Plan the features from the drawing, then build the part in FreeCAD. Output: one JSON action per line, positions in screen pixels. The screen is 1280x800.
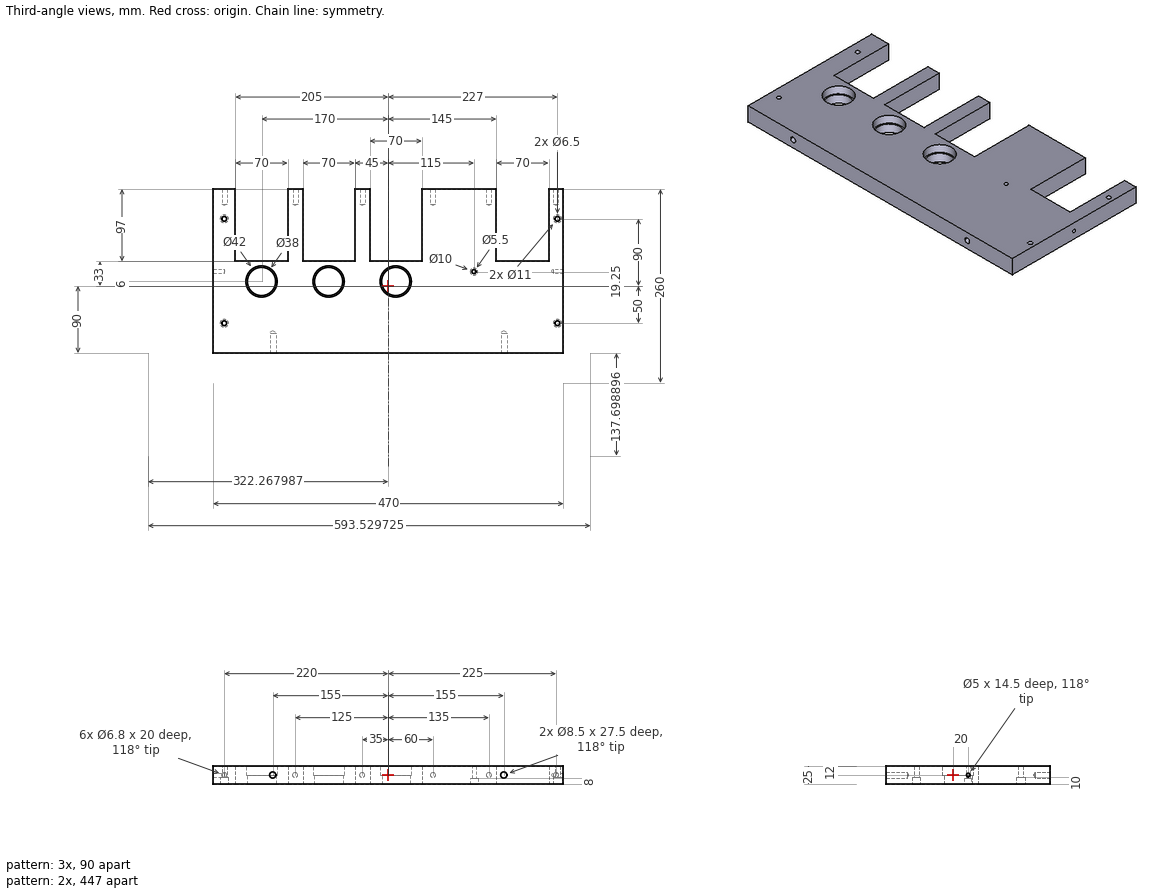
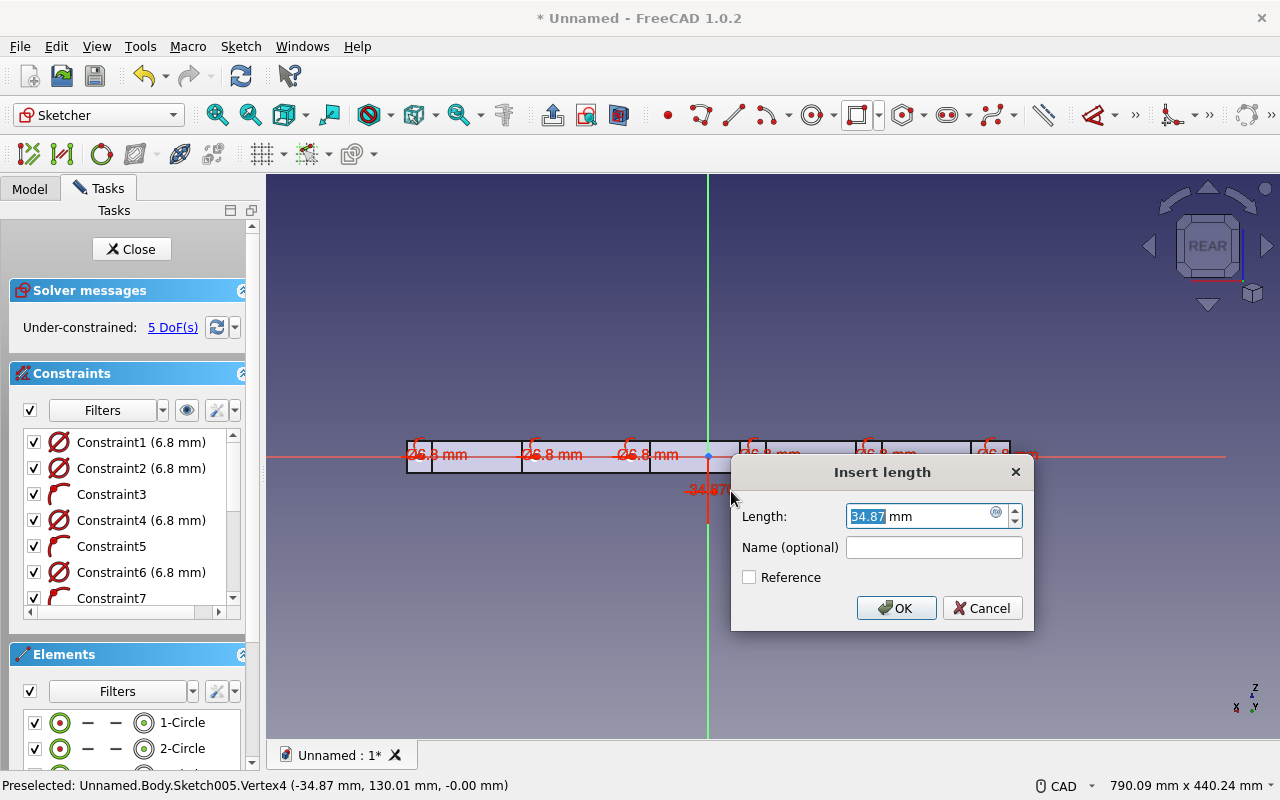
{"action": "type", "text": "35"}
{"action": "key", "text": "Return"}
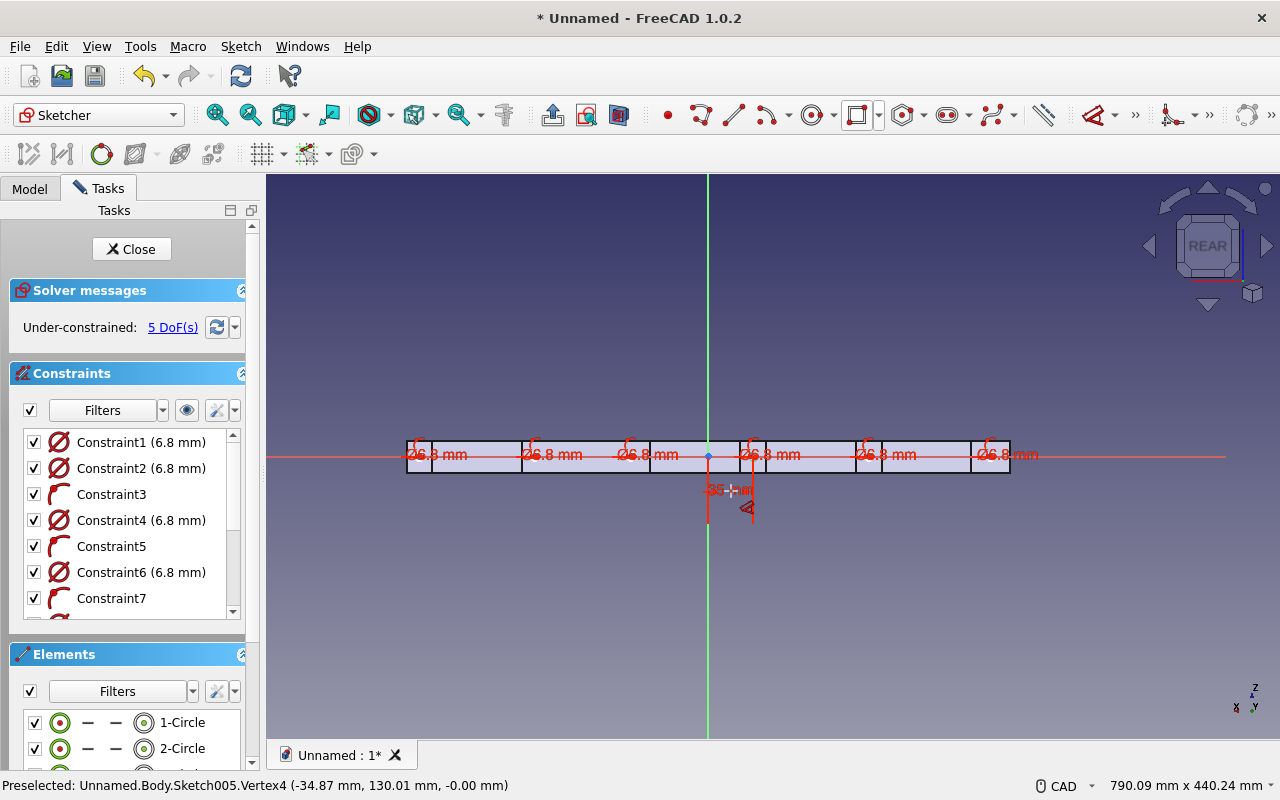
{"action": "left_click", "coordinate": [631, 457]}
{"action": "left_click", "coordinate": [652, 491]}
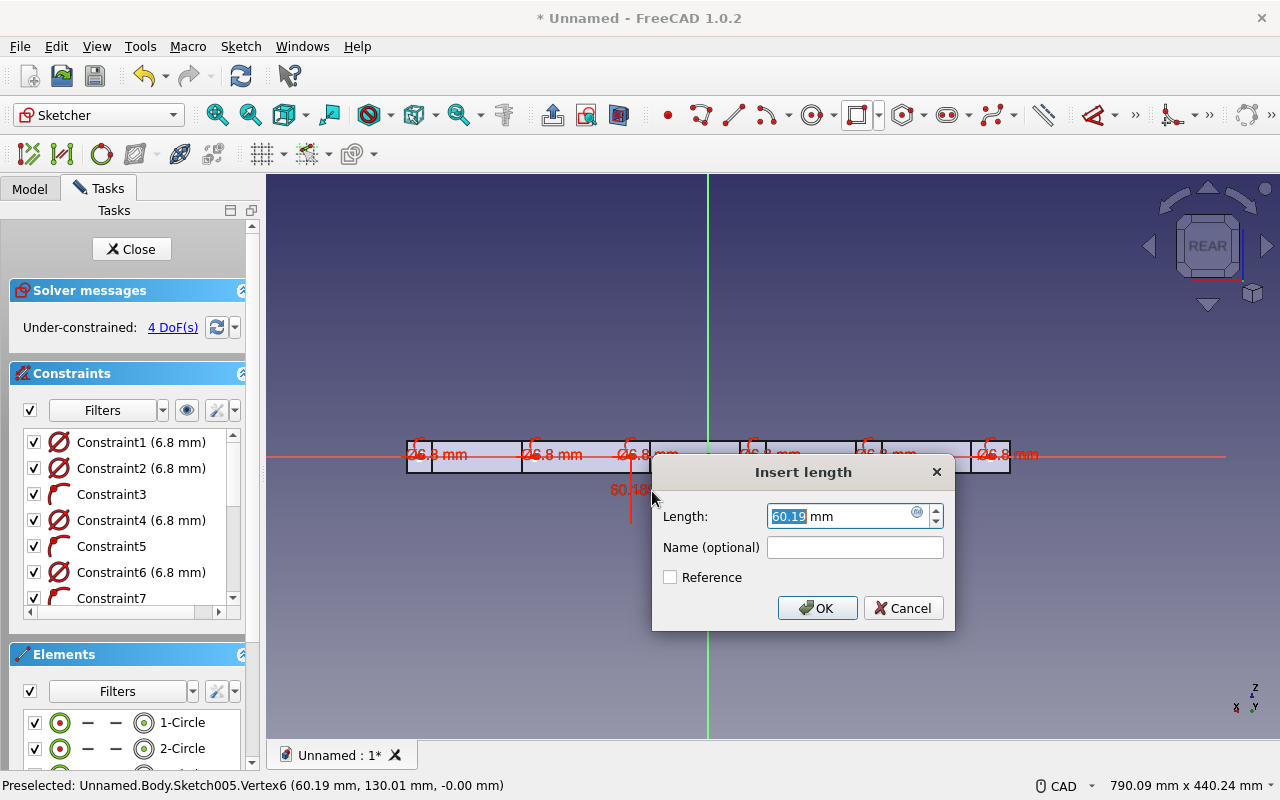
{"action": "type", "text": "60"}
{"action": "key", "text": "Return"}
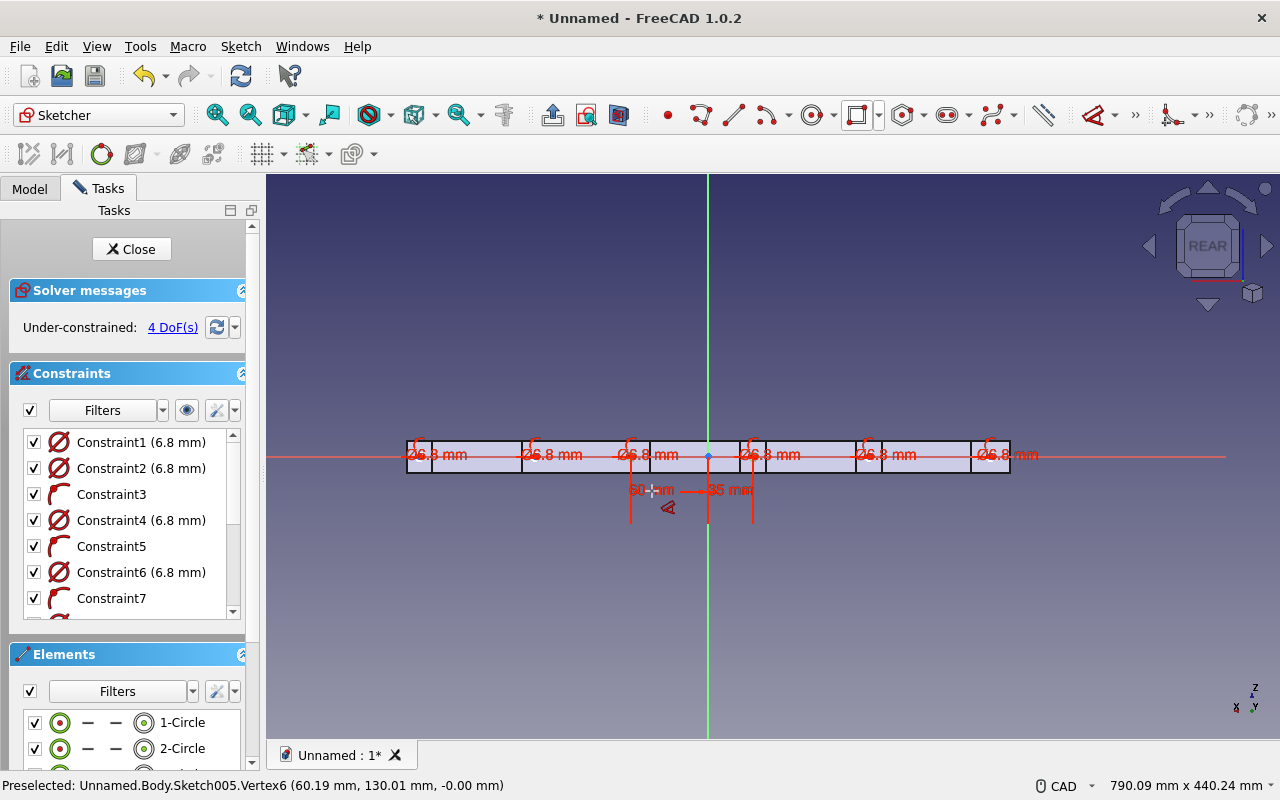
{"action": "left_click", "coordinate": [991, 457]}
{"action": "left_click", "coordinate": [850, 491]}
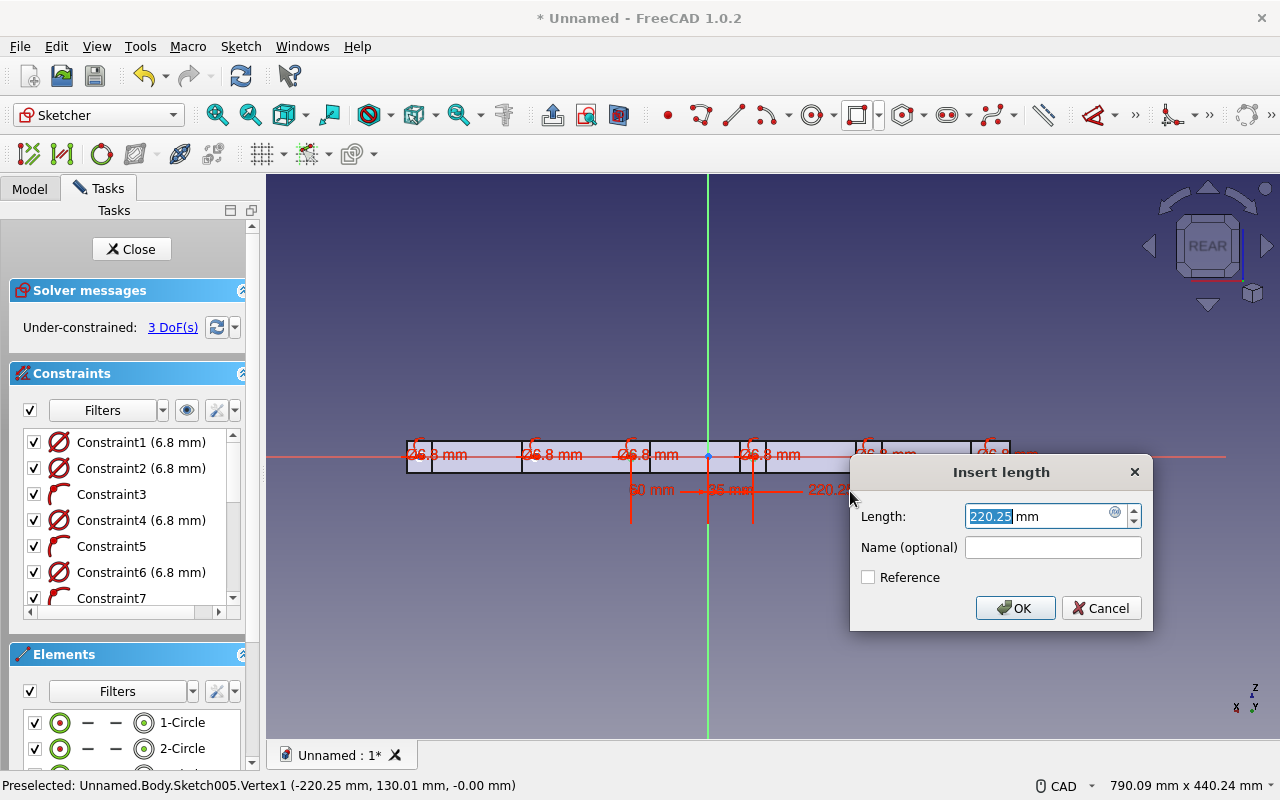
{"action": "type", "text": "220"}
{"action": "key", "text": "Return"}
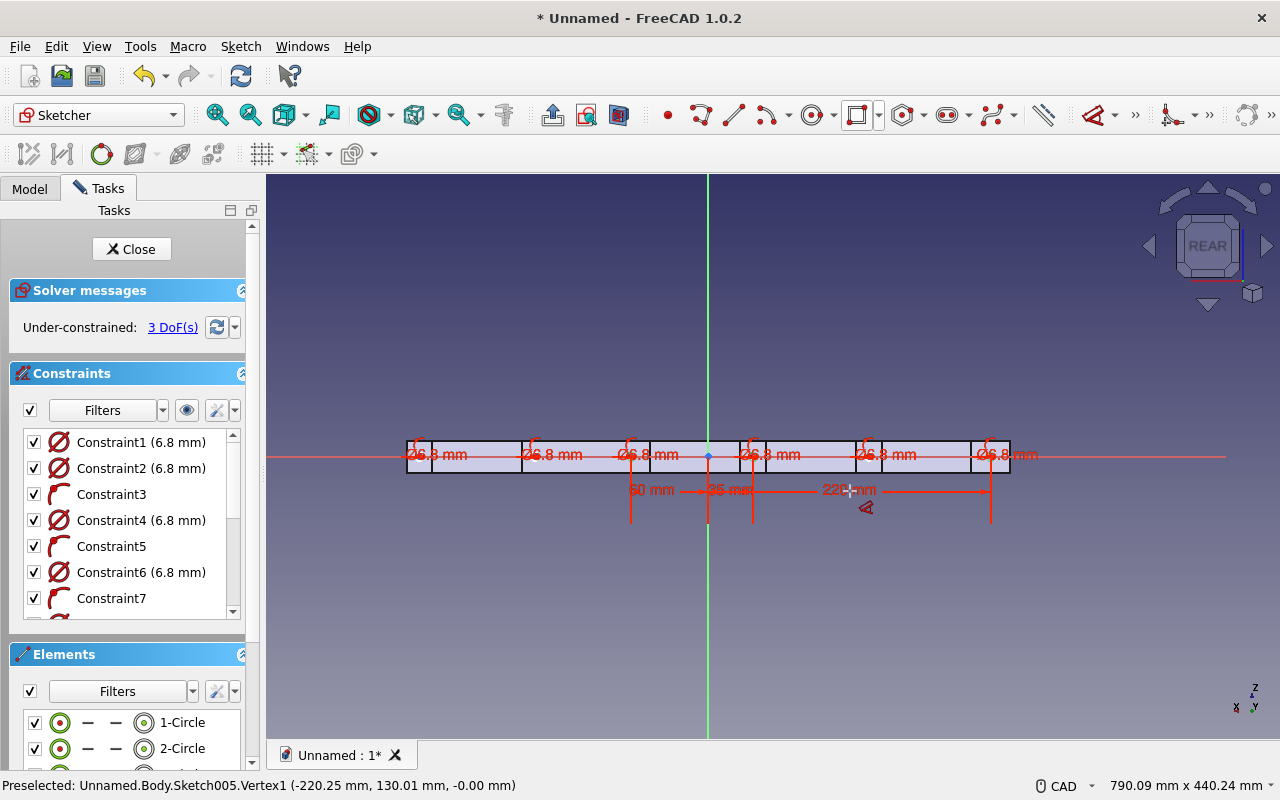
{"action": "left_click", "coordinate": [420, 457]}
{"action": "left_click", "coordinate": [564, 491]}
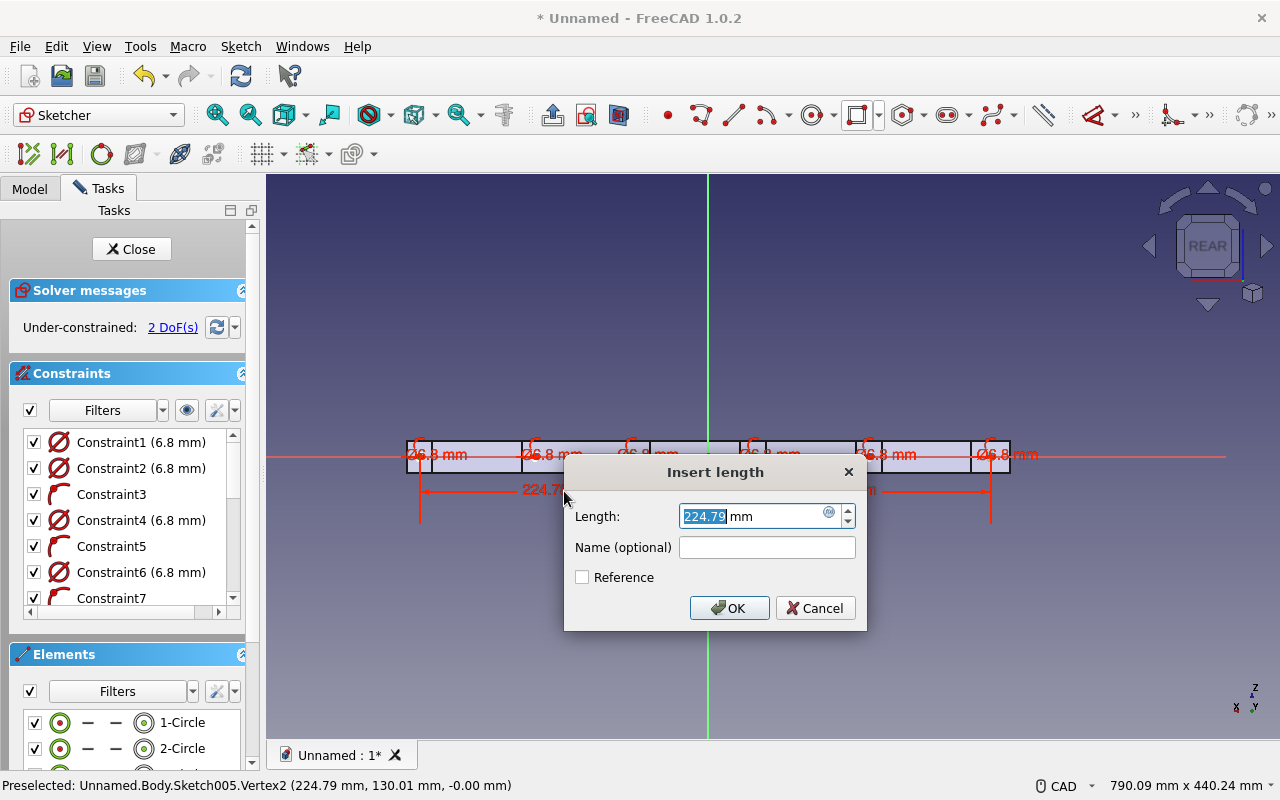
{"action": "type", "text": "225"}
{"action": "key", "text": "Return"}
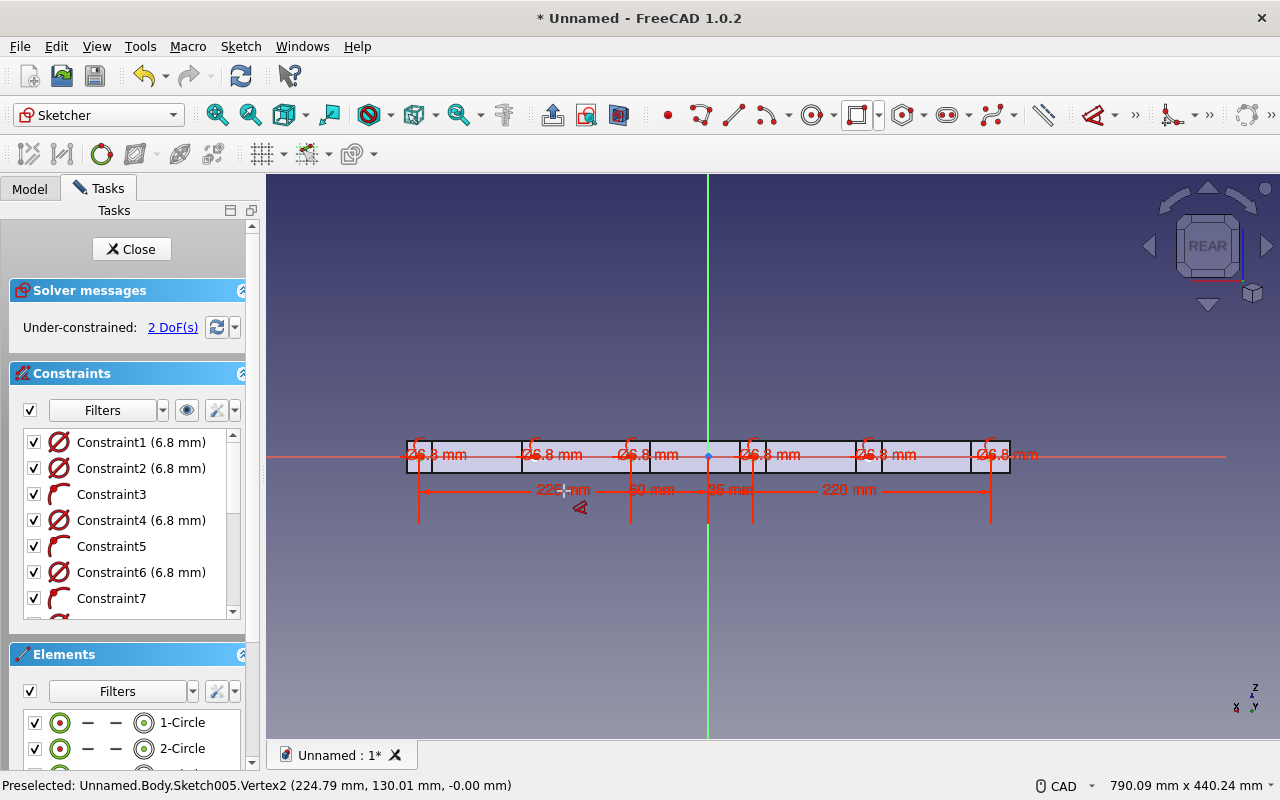
{"action": "left_click", "coordinate": [535, 457]}
{"action": "left_click", "coordinate": [622, 423]}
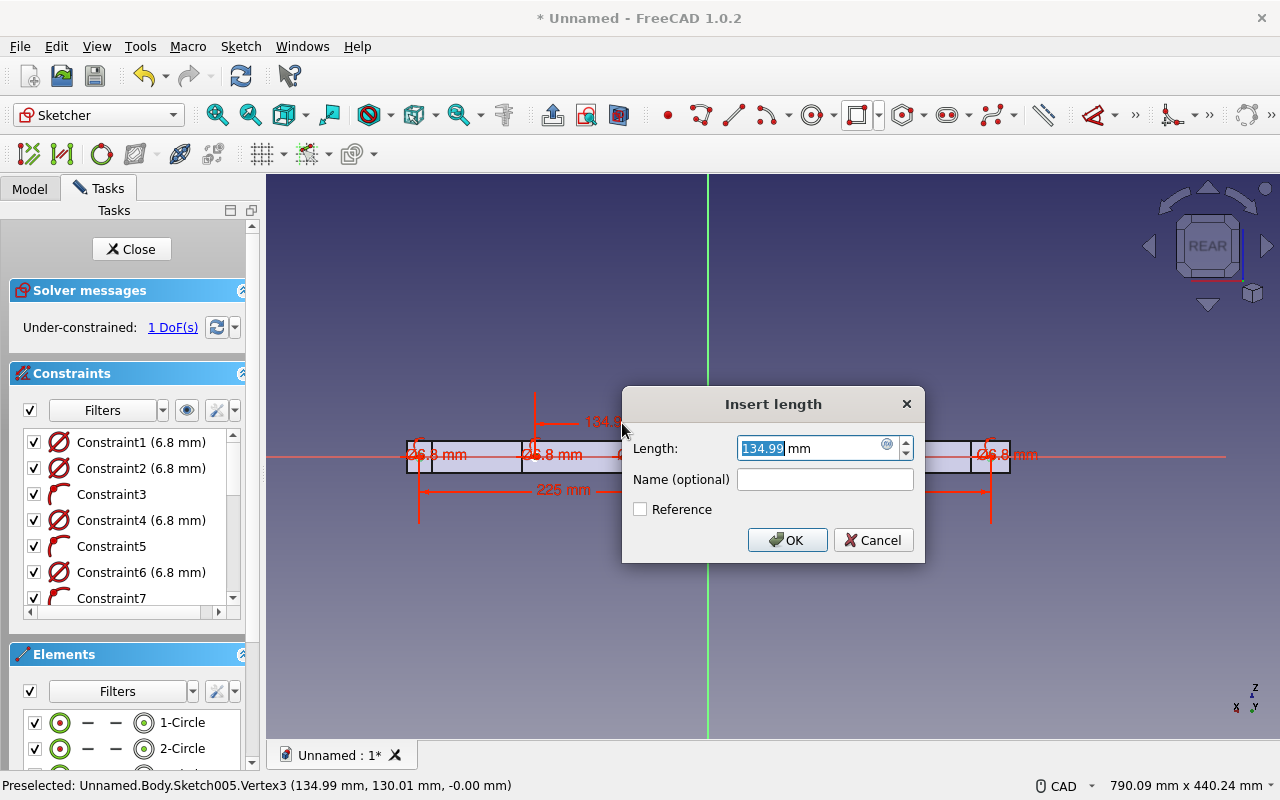
{"action": "type", "text": "135"}
{"action": "key", "text": "Return"}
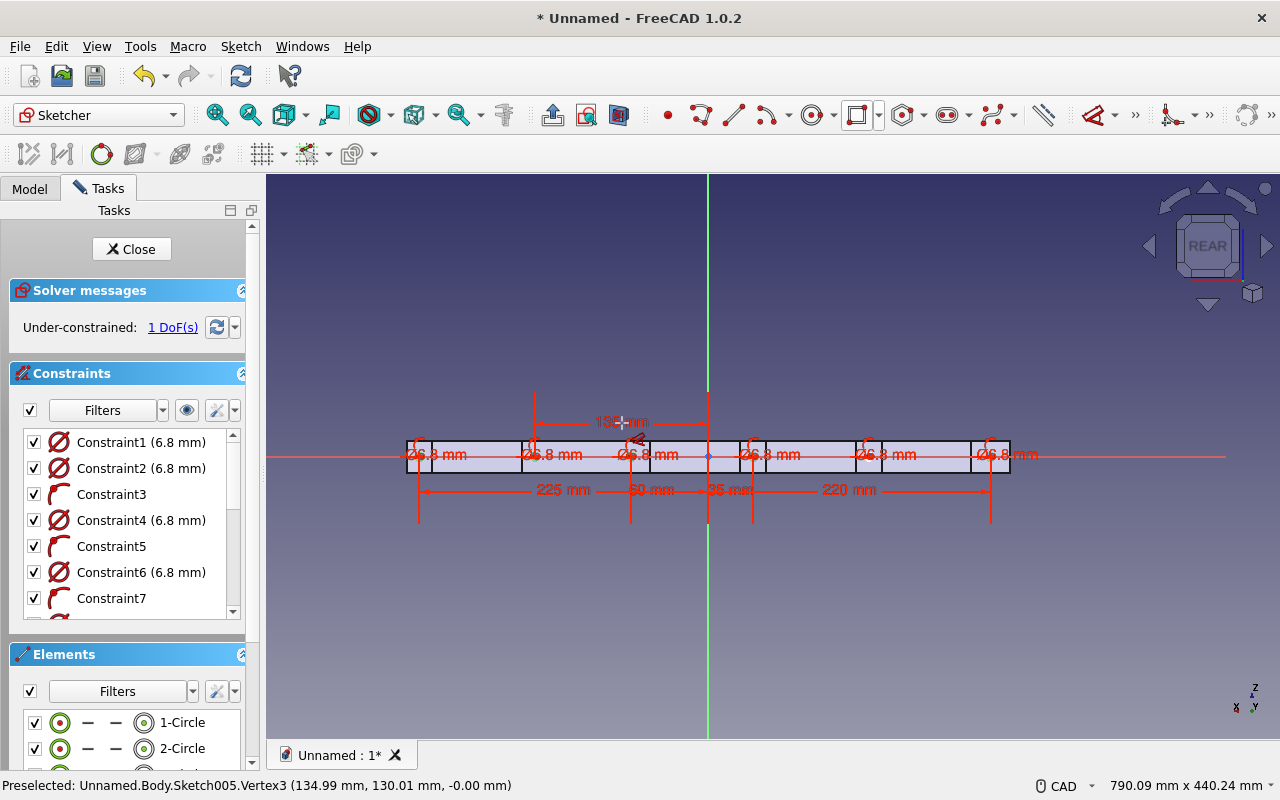
{"action": "left_click", "coordinate": [869, 457]}
{"action": "left_click", "coordinate": [789, 423]}